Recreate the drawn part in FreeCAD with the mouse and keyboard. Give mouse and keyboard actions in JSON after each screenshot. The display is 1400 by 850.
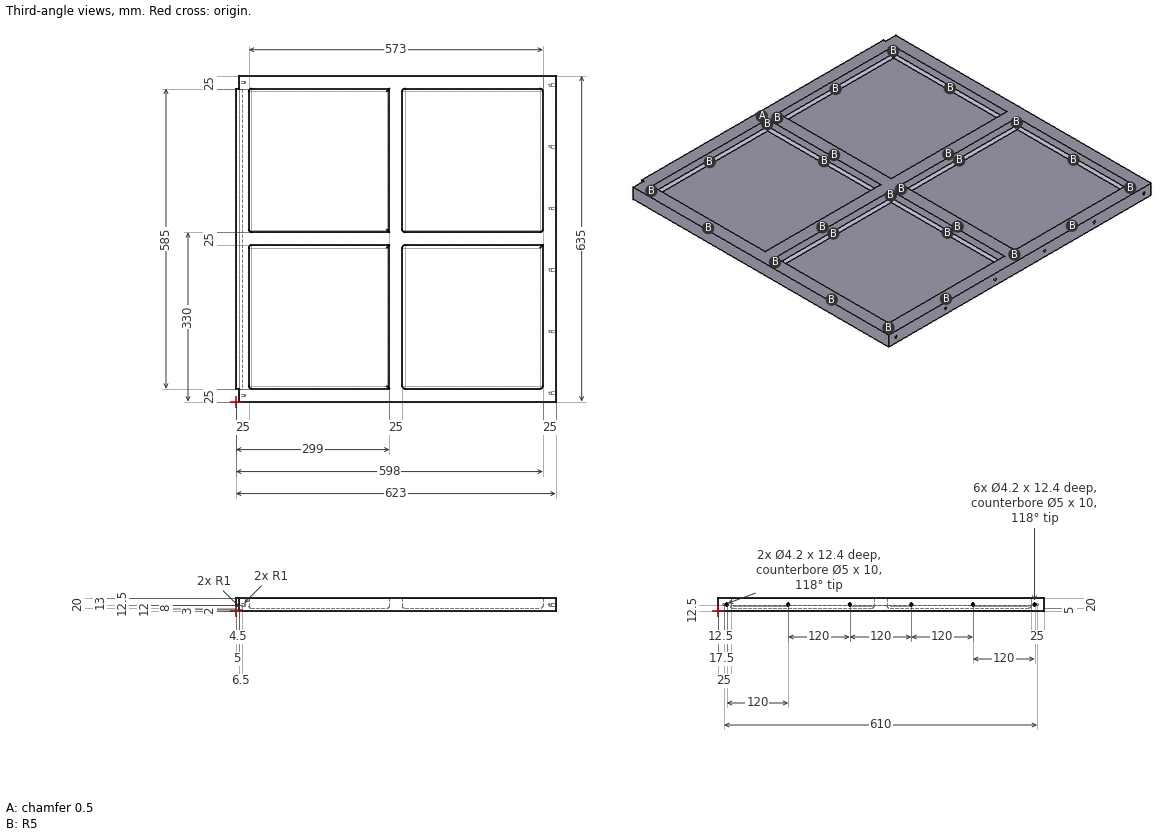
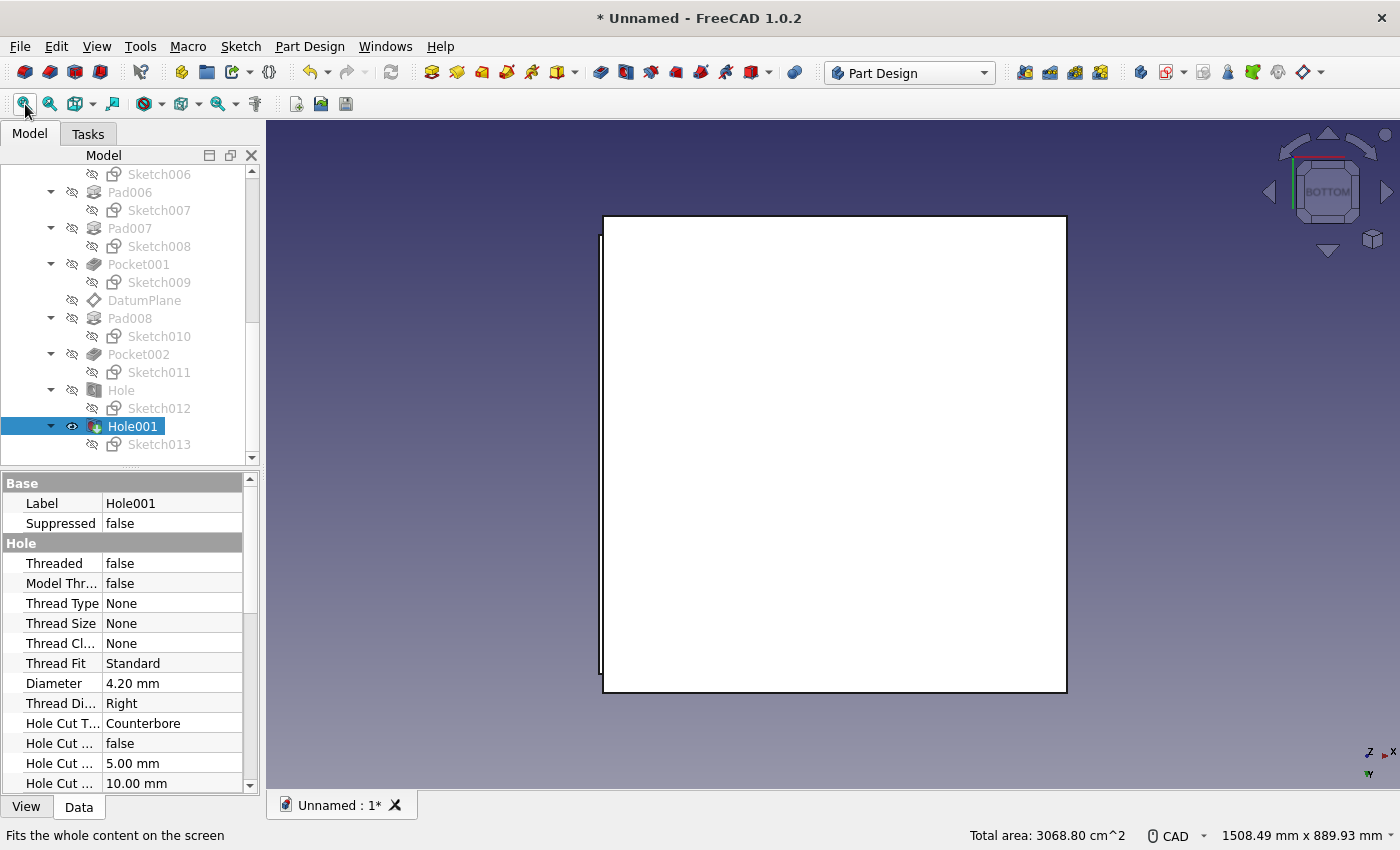
{"action": "scroll", "coordinate": [1048, 234], "scroll_direction": "up", "scroll_amount": 5}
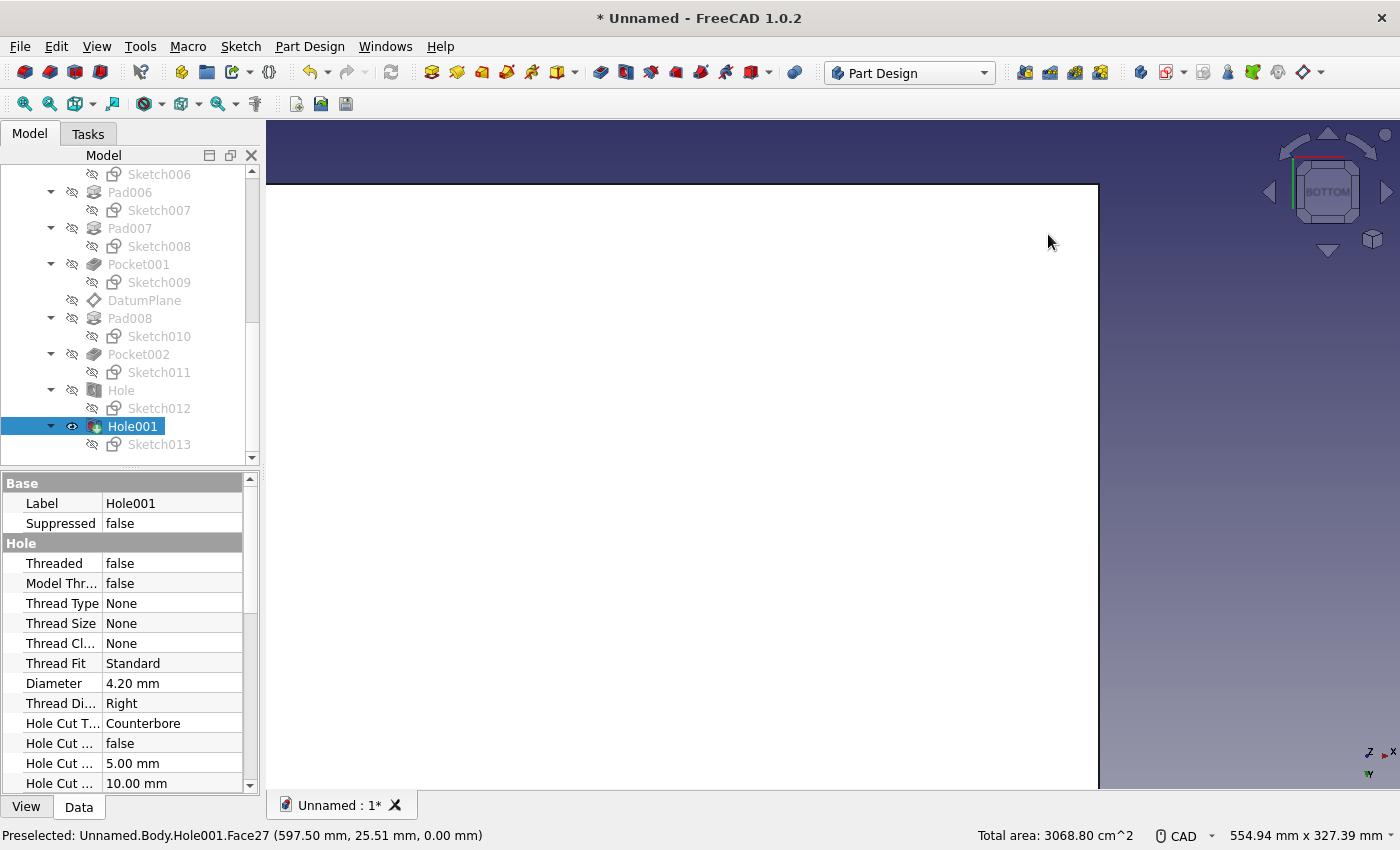
{"action": "left_click", "coordinate": [25, 104]}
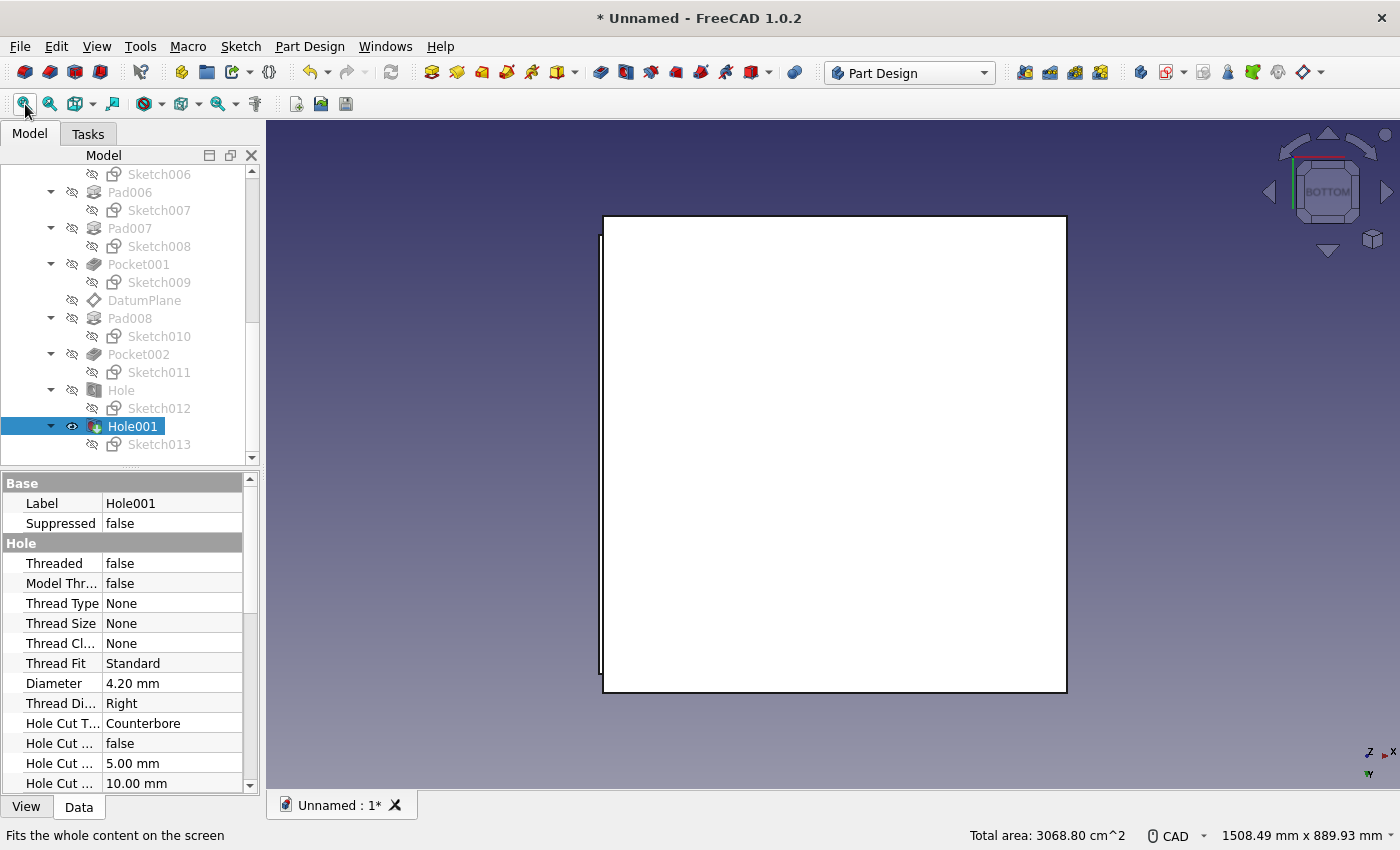
{"action": "key", "text": "4"}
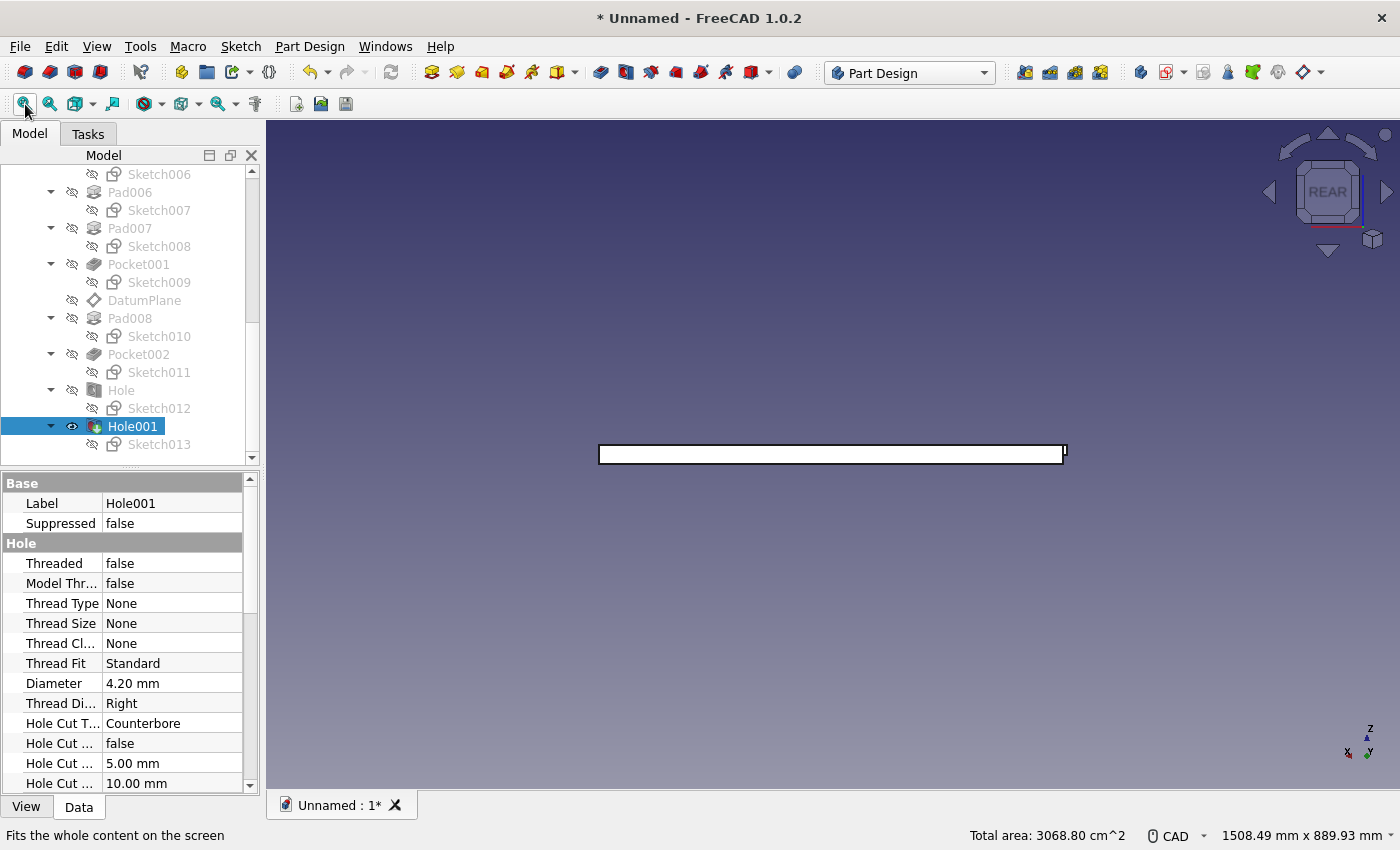
{"action": "left_click", "coordinate": [25, 104]}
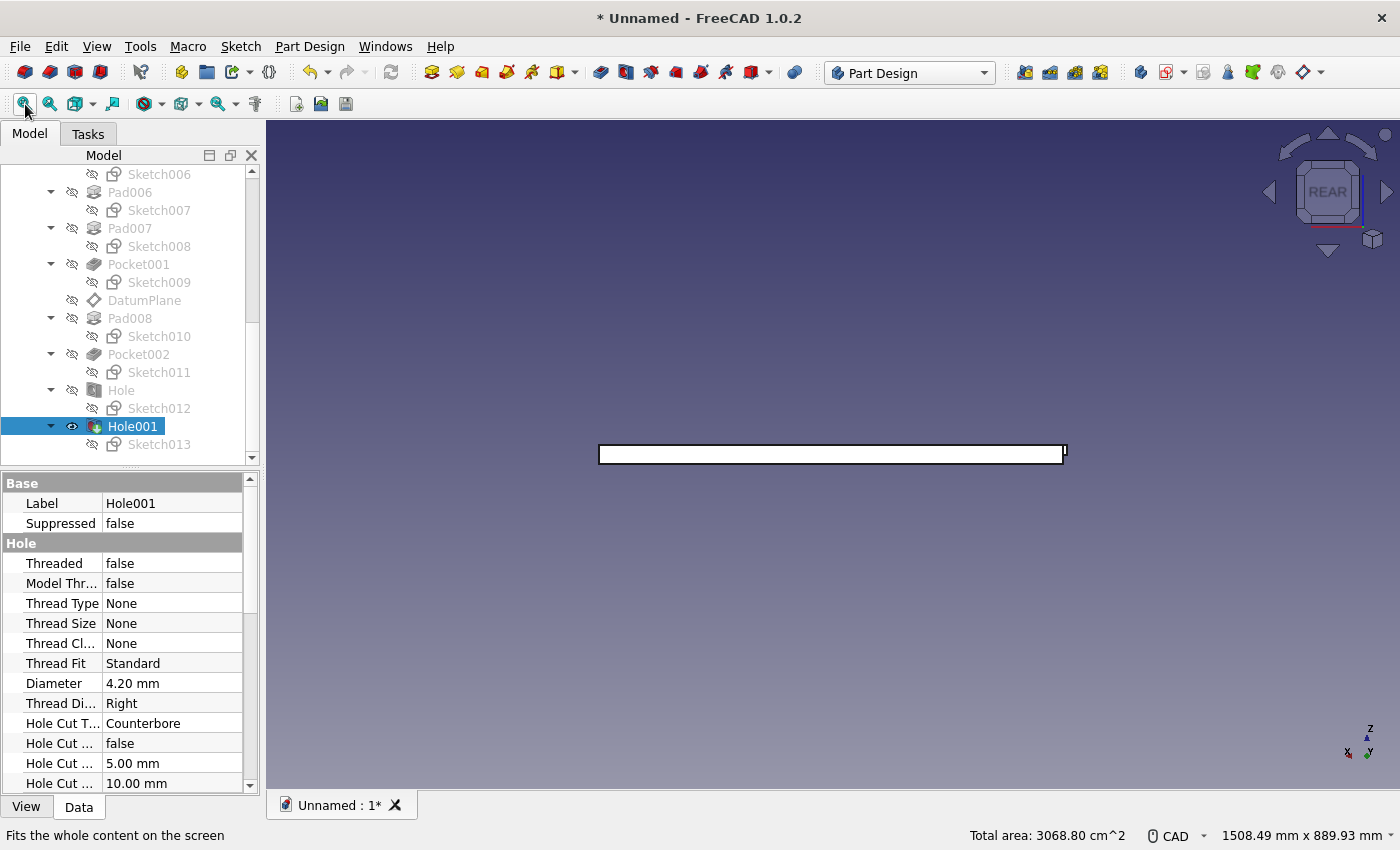
{"action": "scroll", "coordinate": [618, 452], "scroll_direction": "up", "scroll_amount": 5}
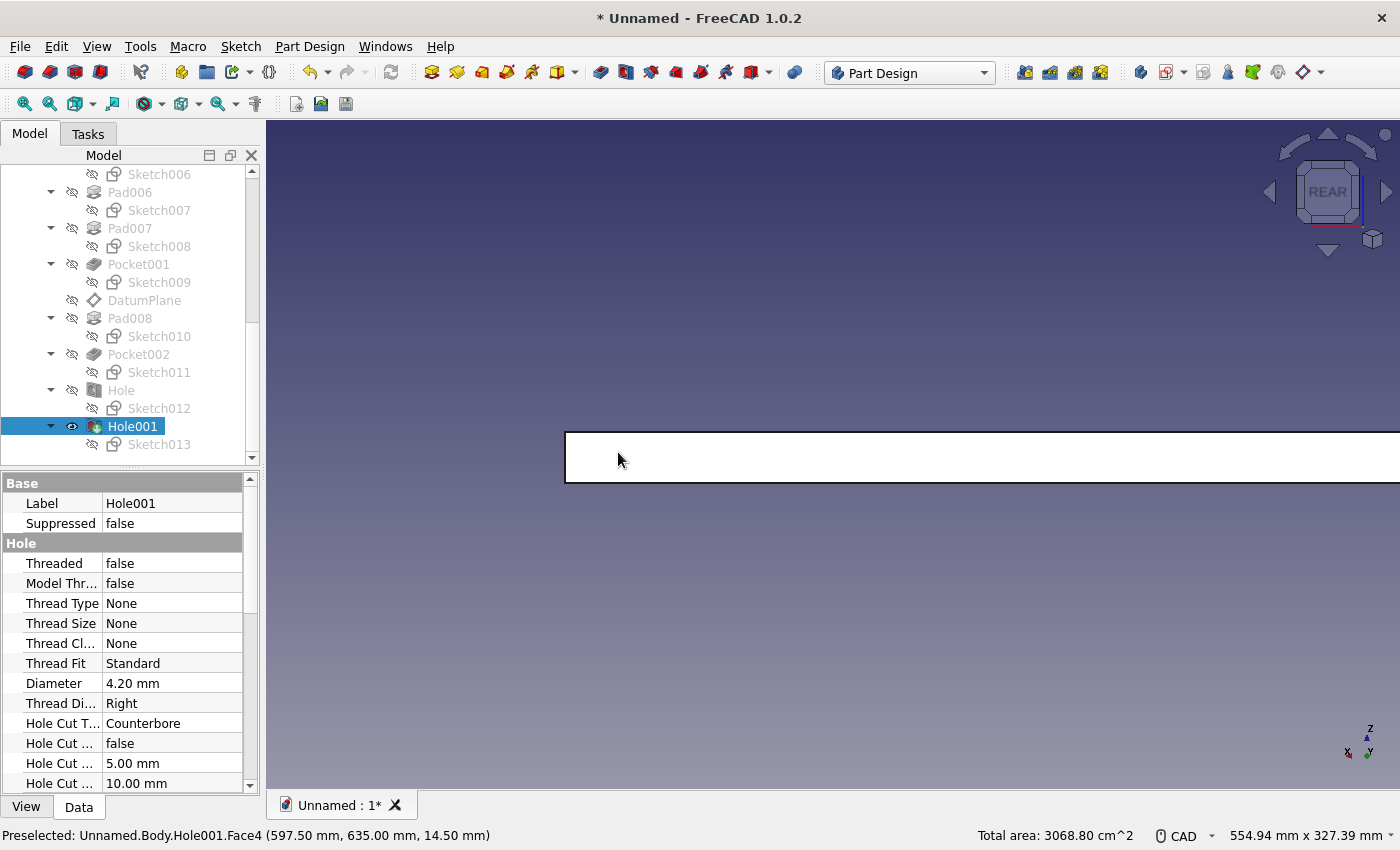
{"action": "left_click", "coordinate": [25, 104]}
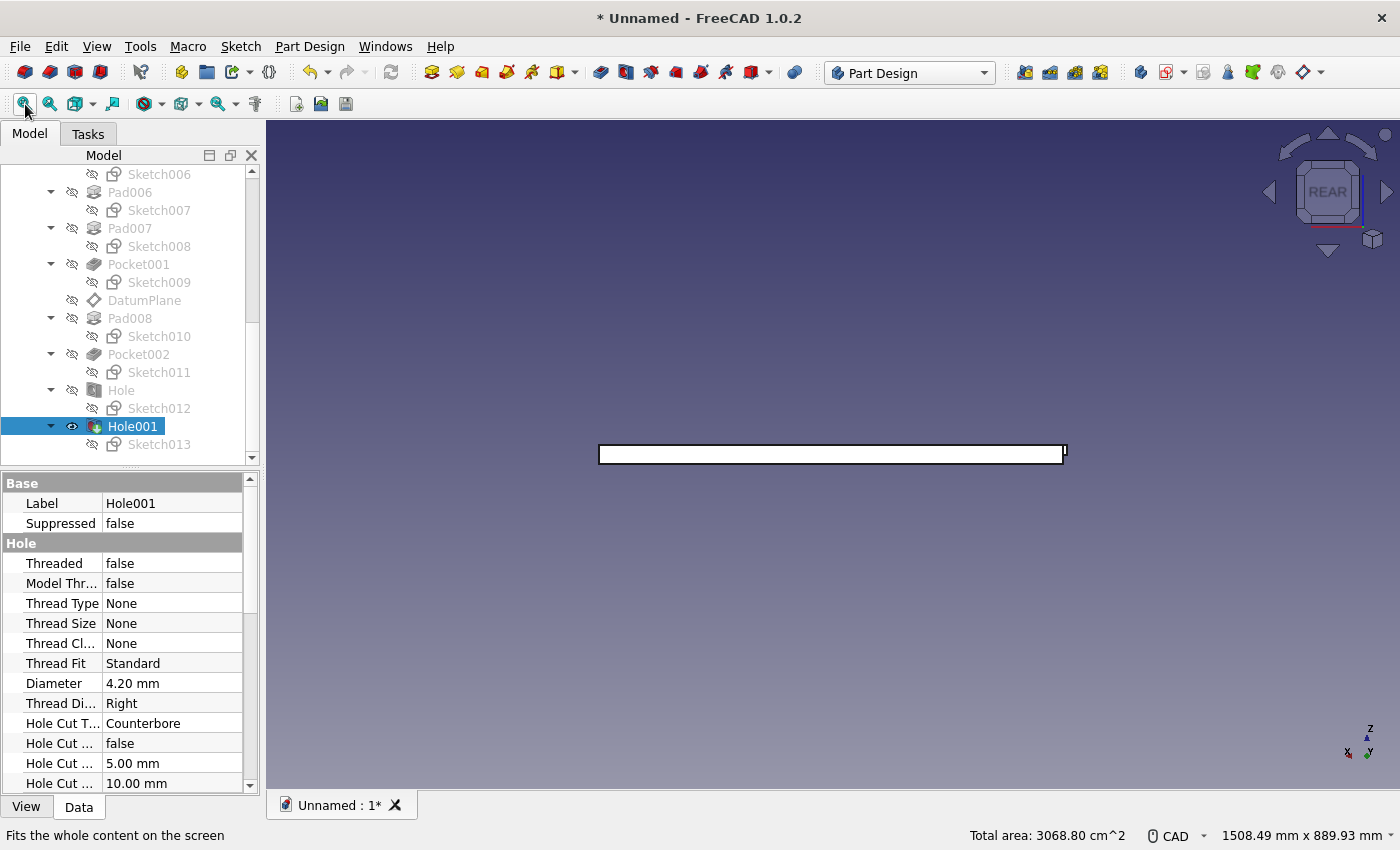
{"action": "key", "text": "6"}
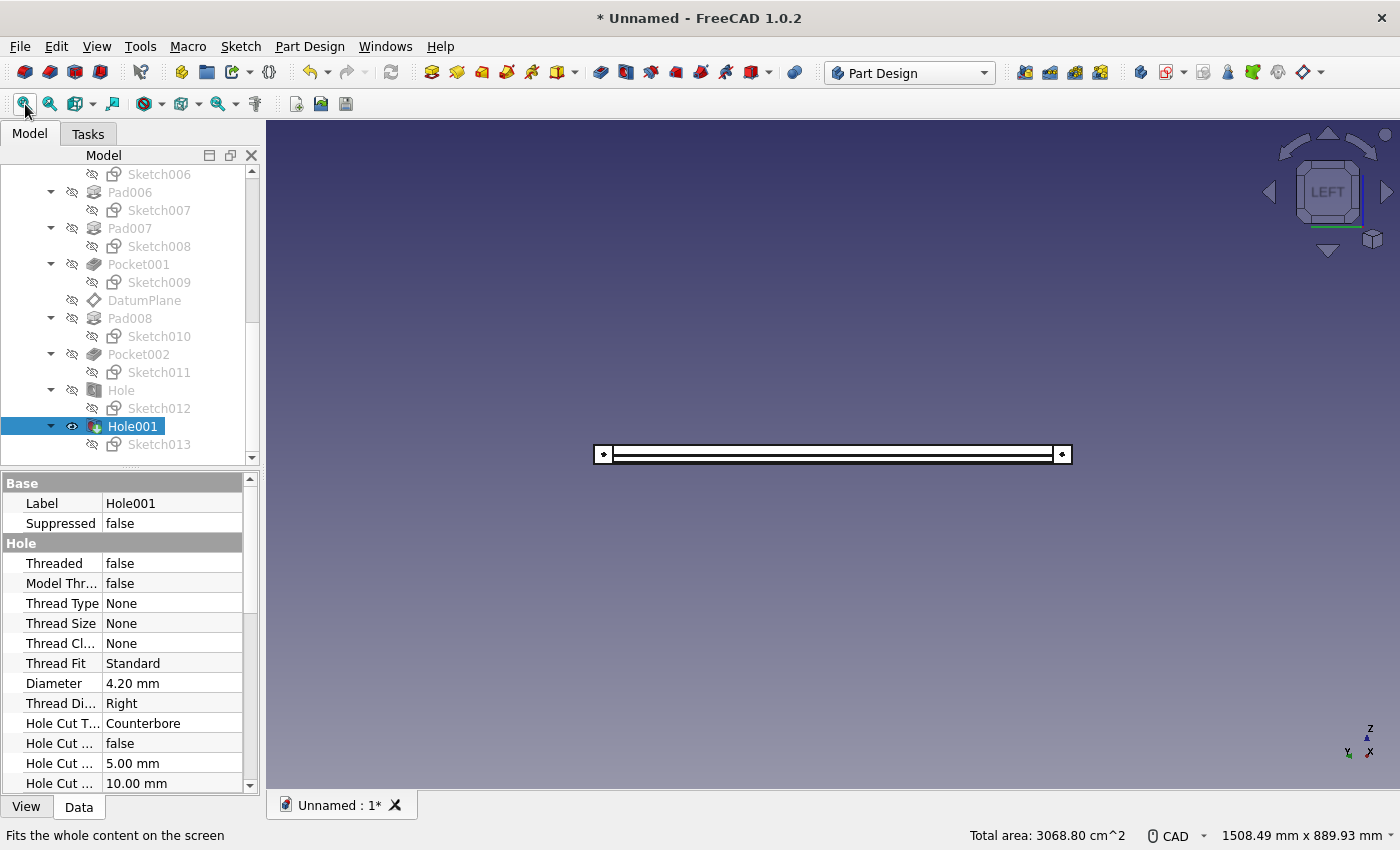
{"action": "left_click", "coordinate": [25, 104]}